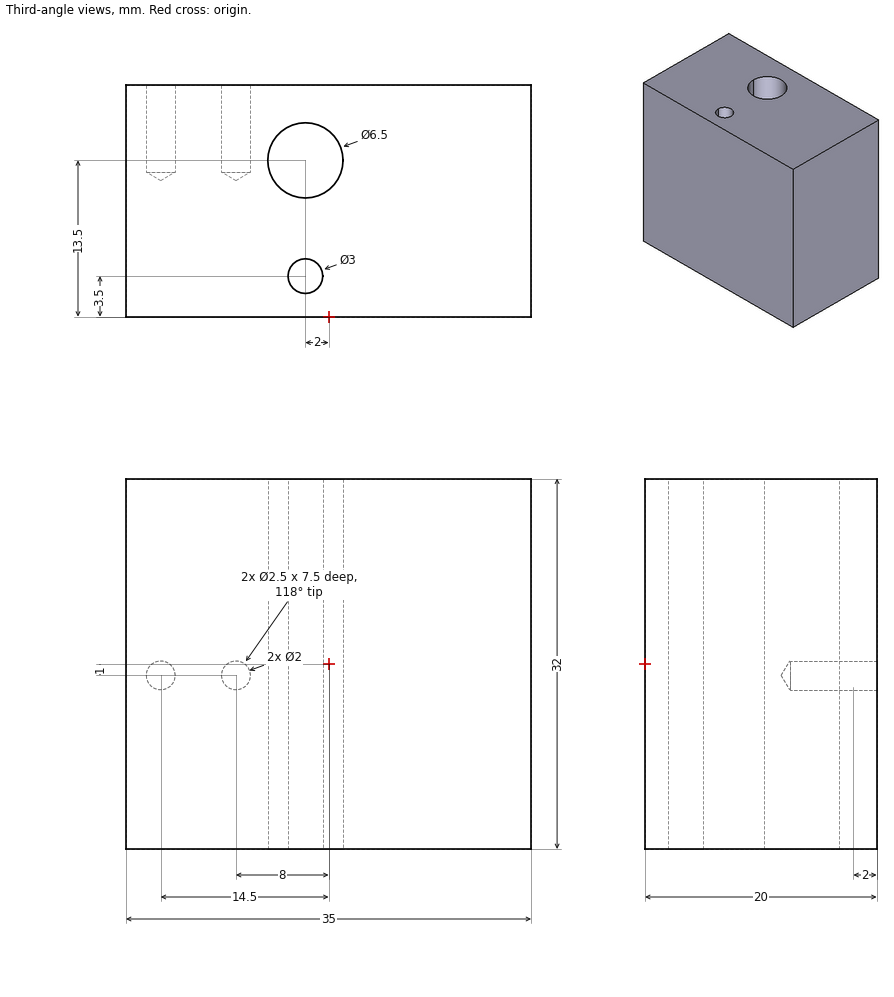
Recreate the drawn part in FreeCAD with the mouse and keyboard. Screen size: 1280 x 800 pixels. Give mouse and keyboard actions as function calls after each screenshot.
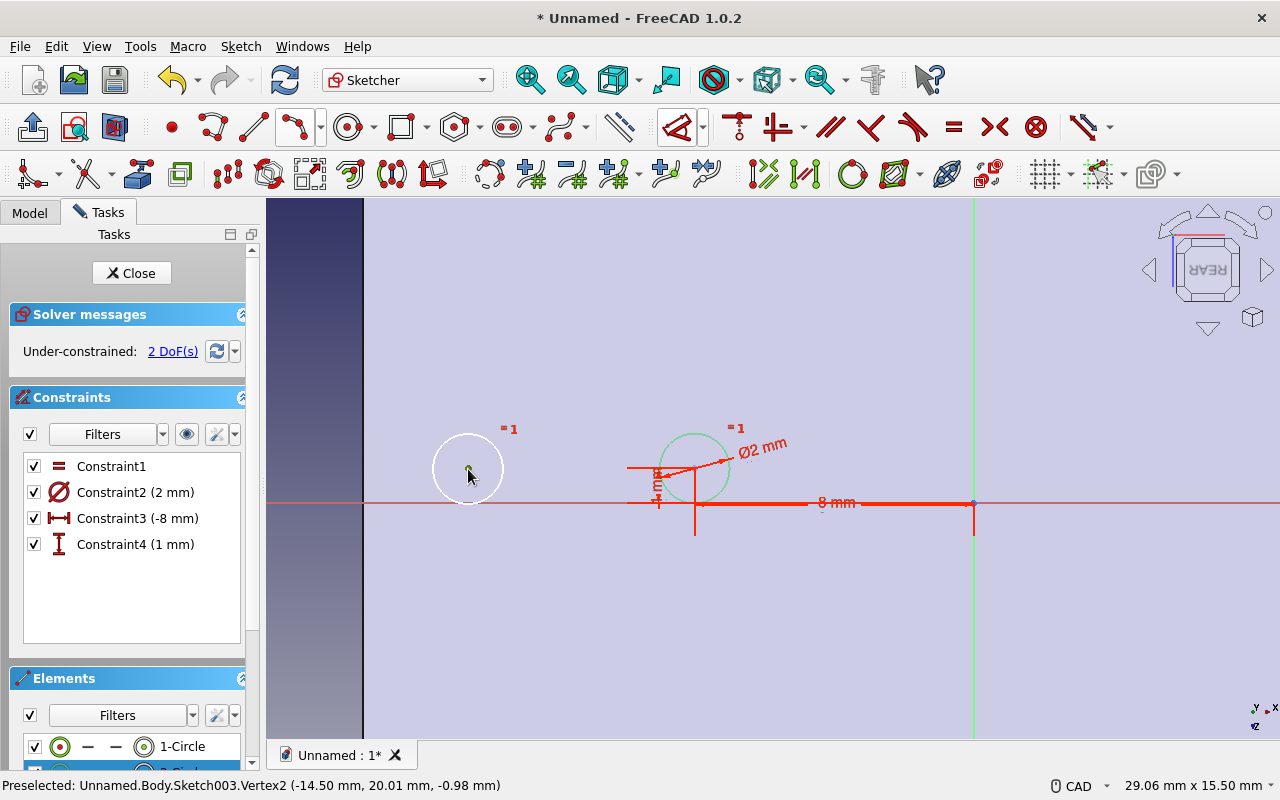
key(i)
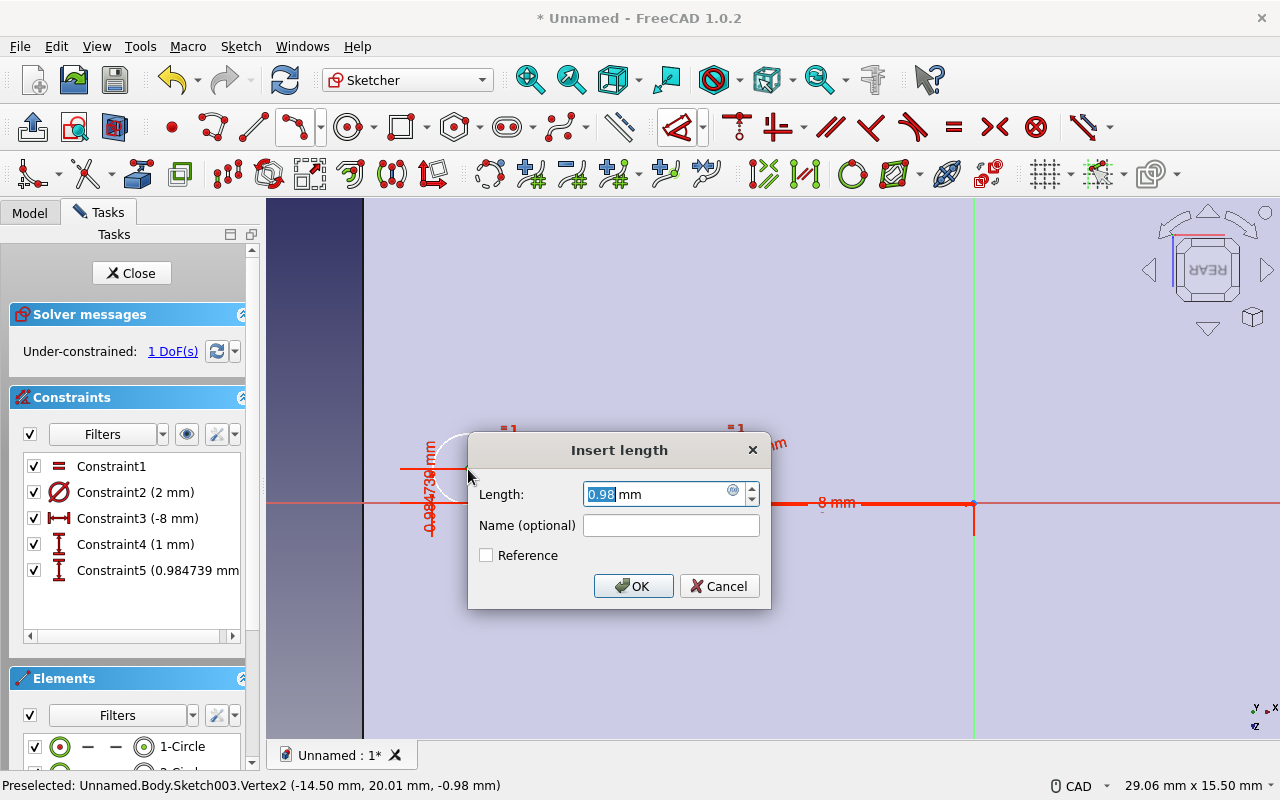
text(1)
key(Return)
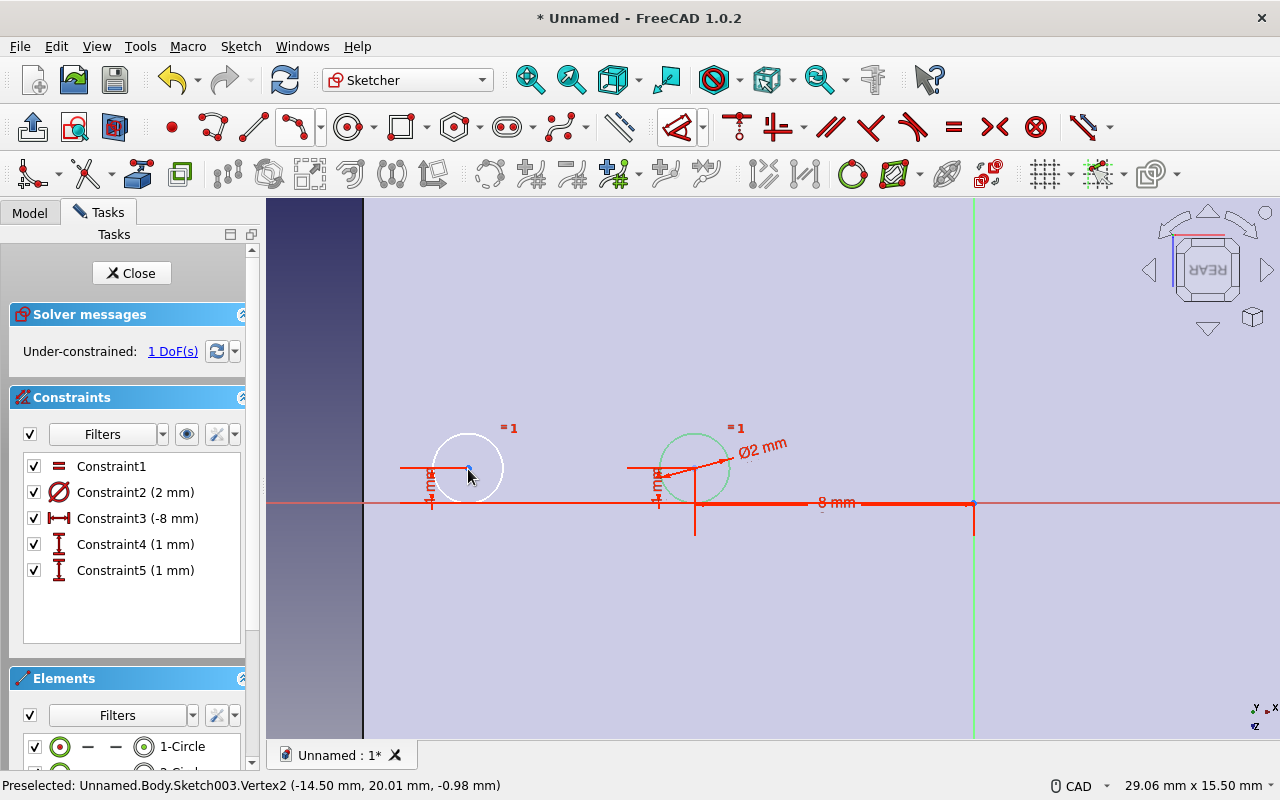
click(468, 468)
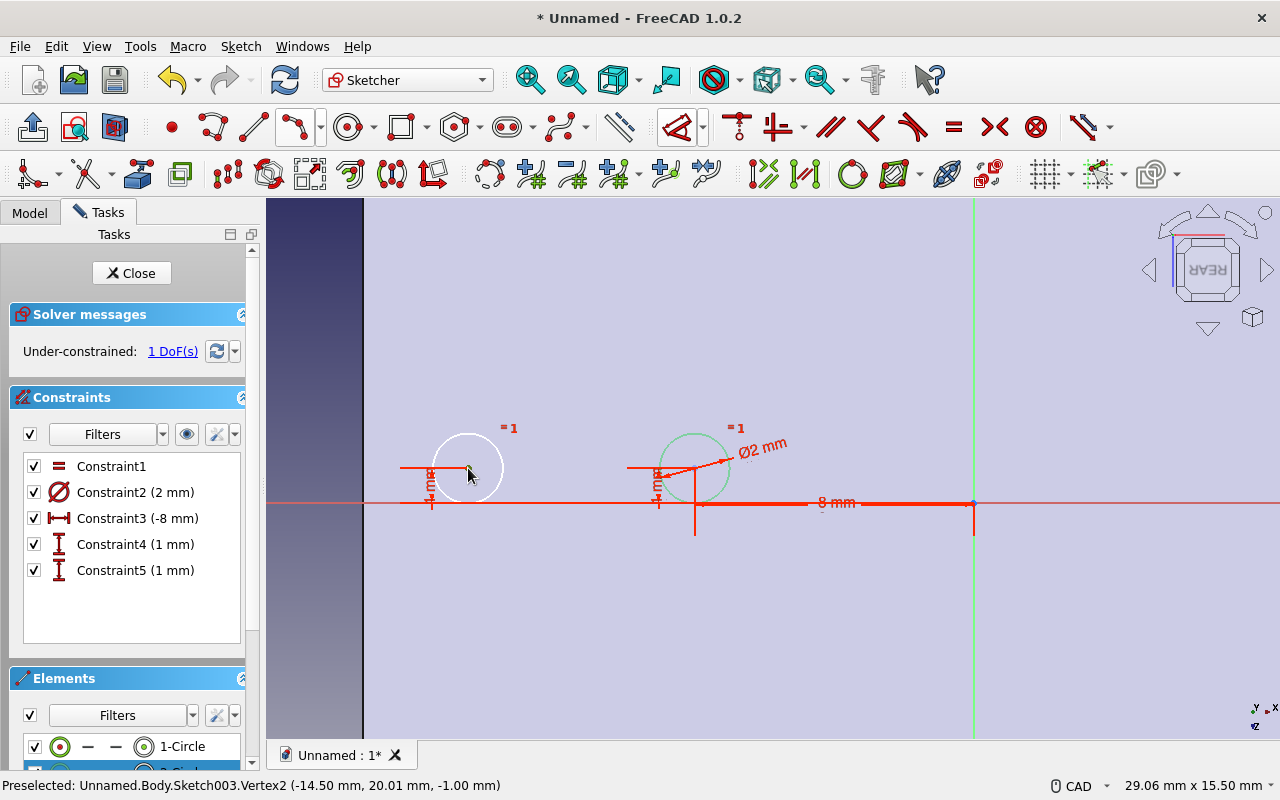
key(l)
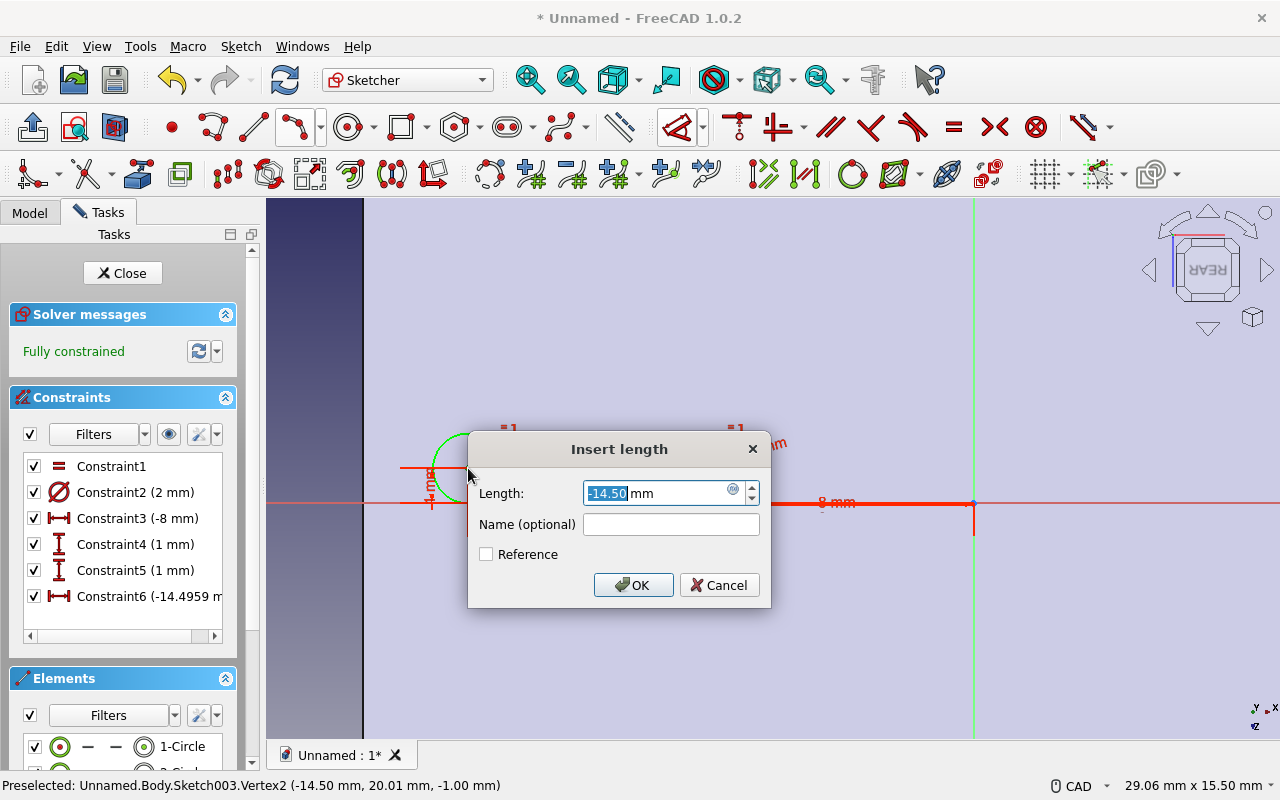
text(-14.5)
key(Return)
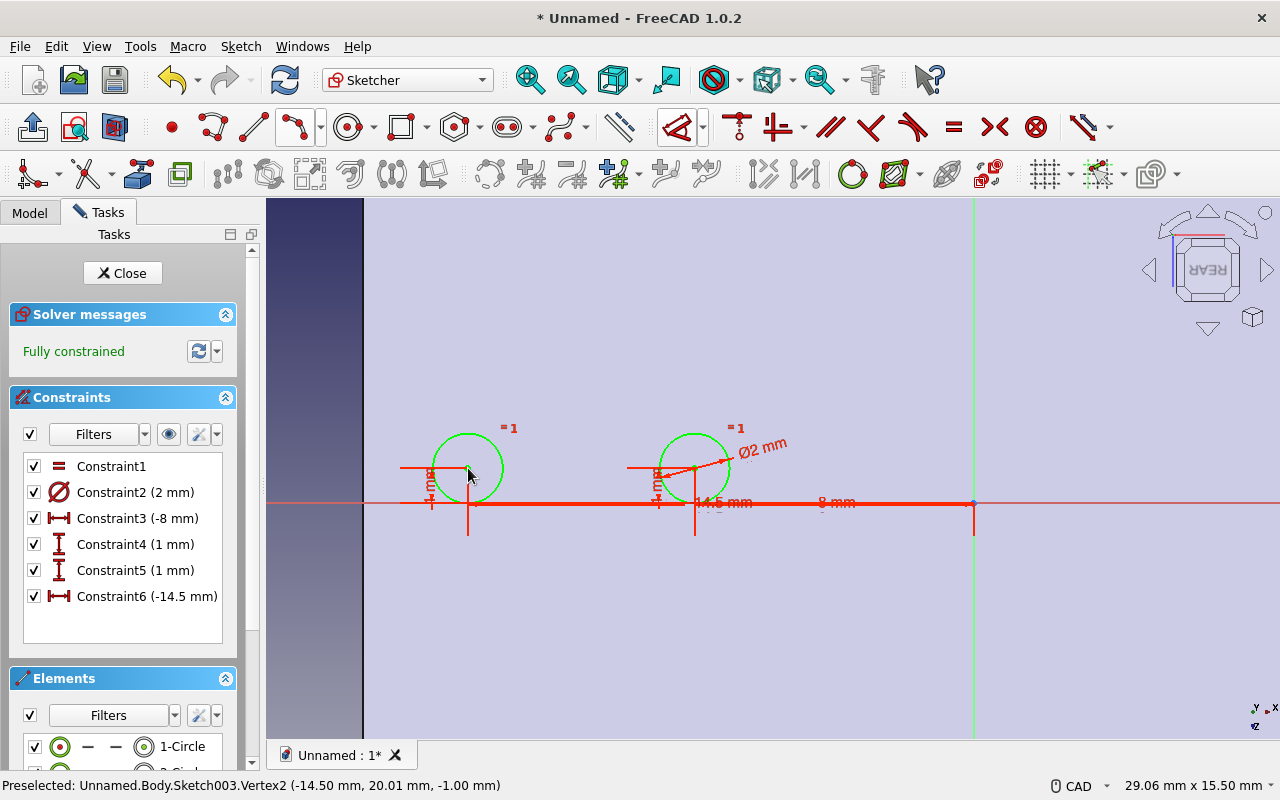
click(123, 273)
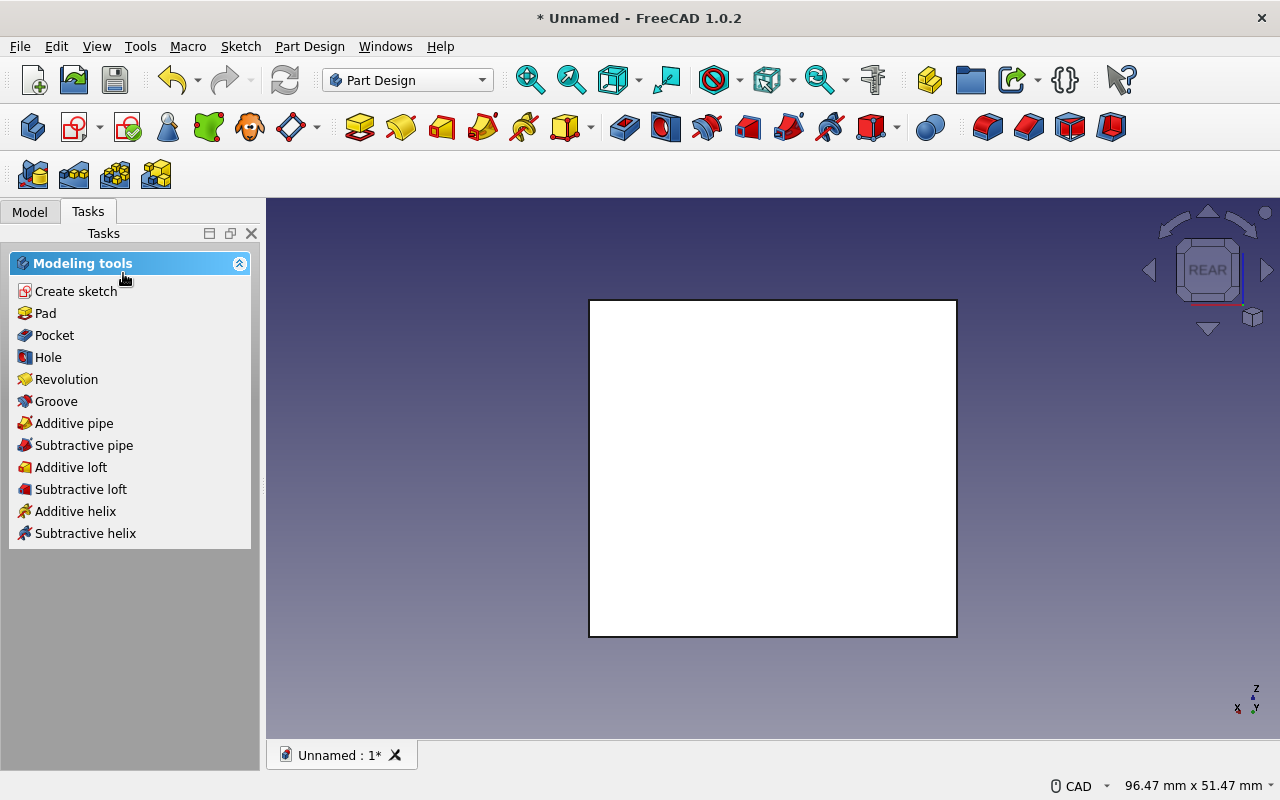
click(625, 128)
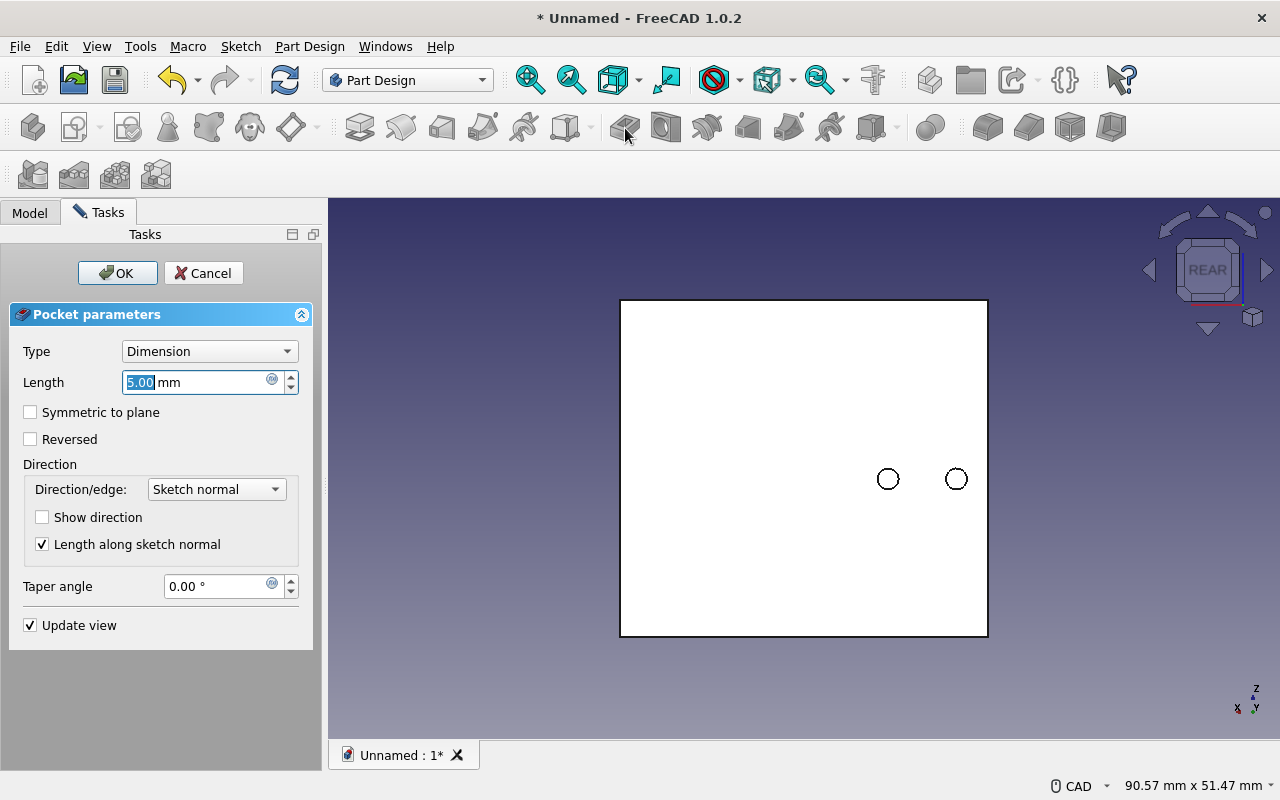
text(2)
key(Tab)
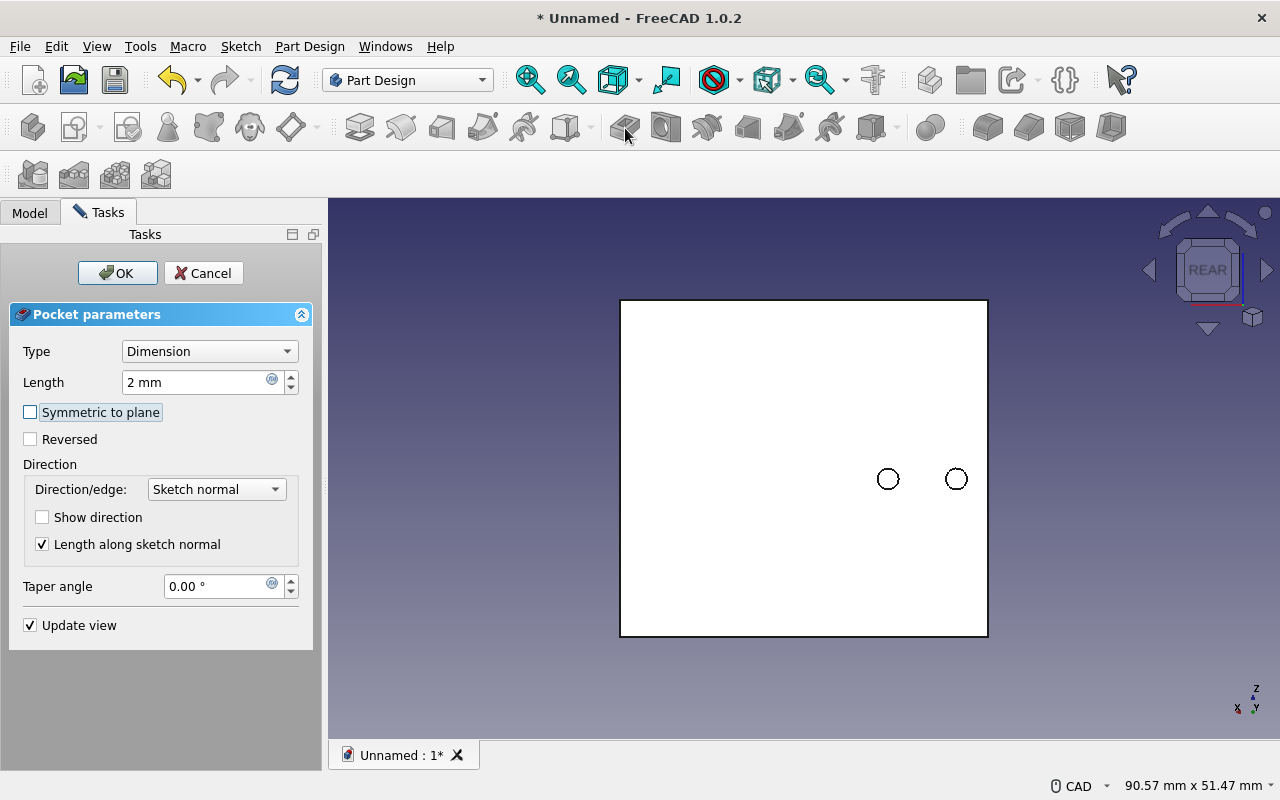
click(118, 273)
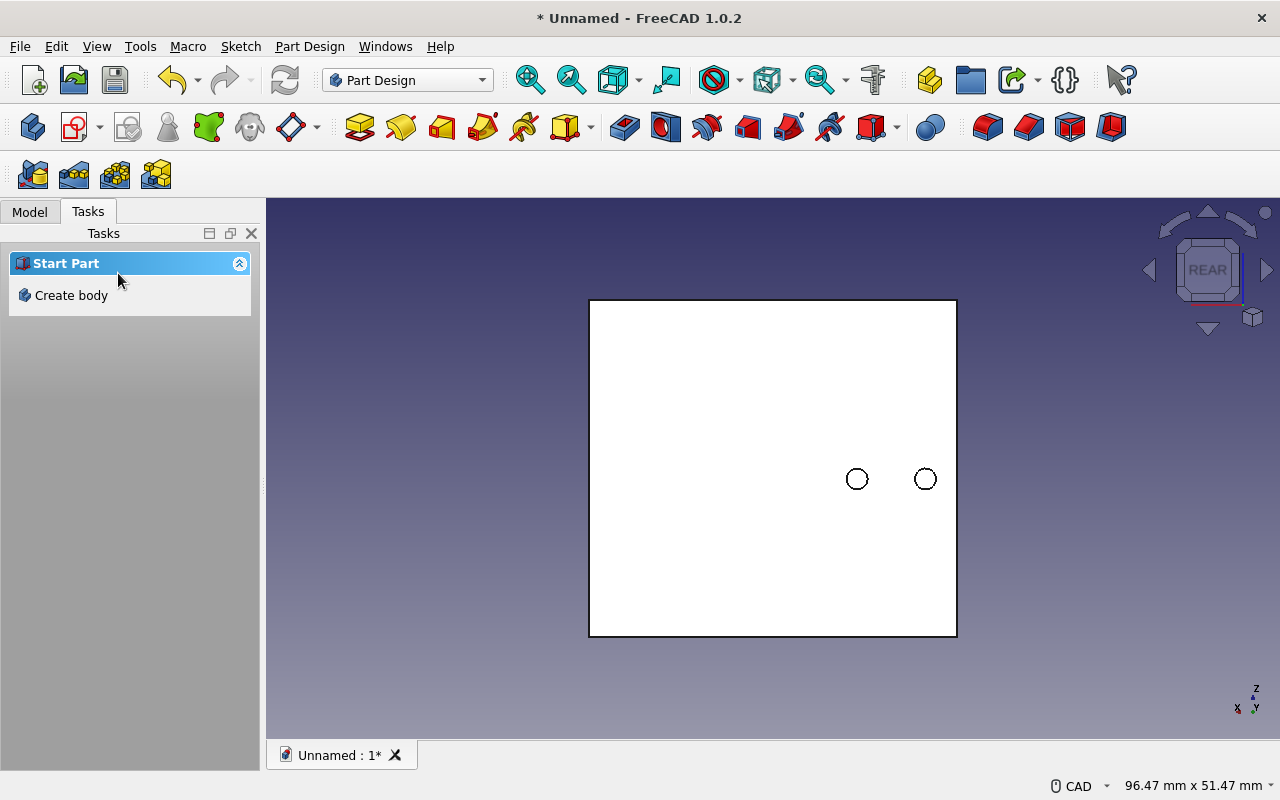
click(720, 468)